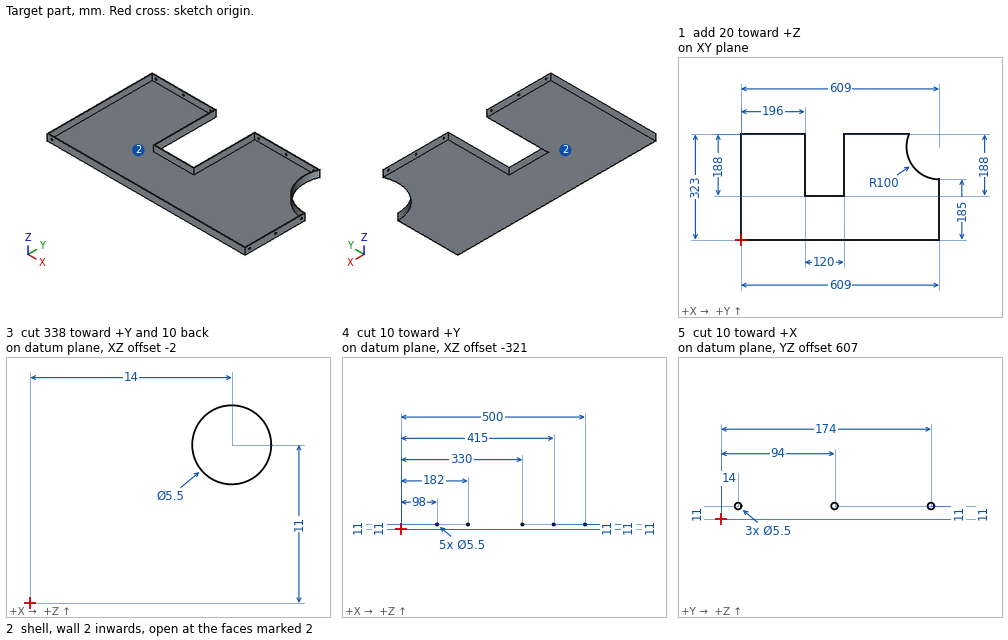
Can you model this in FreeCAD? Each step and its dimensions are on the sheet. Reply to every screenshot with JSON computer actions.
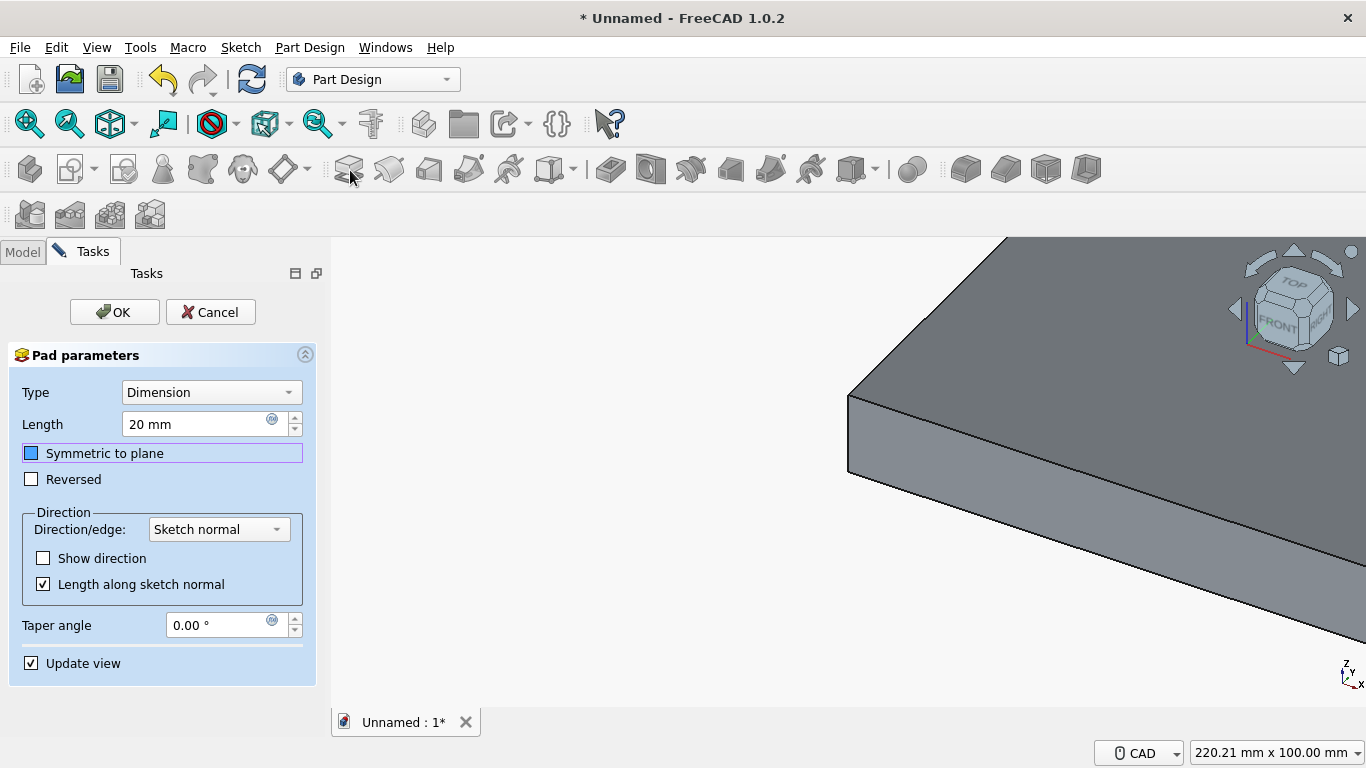
{"action": "left_click", "coordinate": [115, 312]}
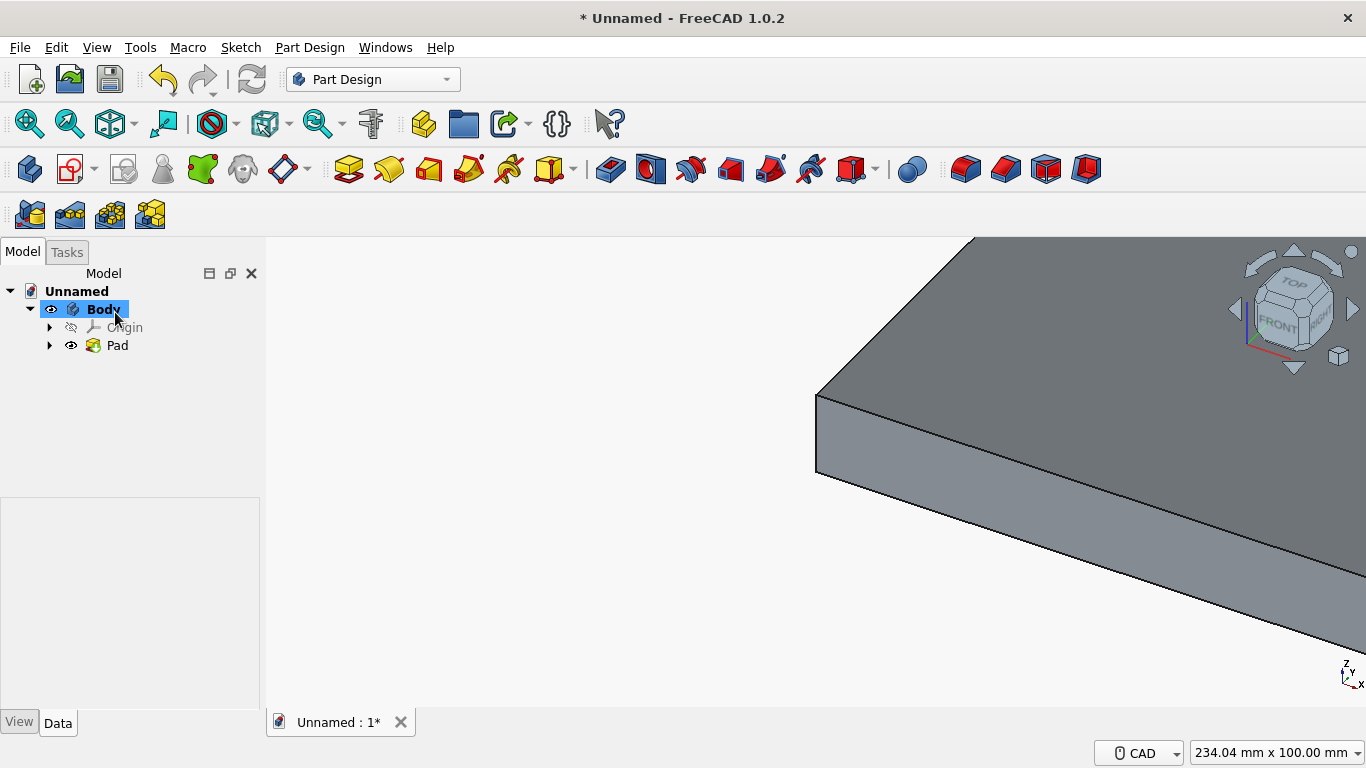
{"action": "left_click", "coordinate": [30, 124]}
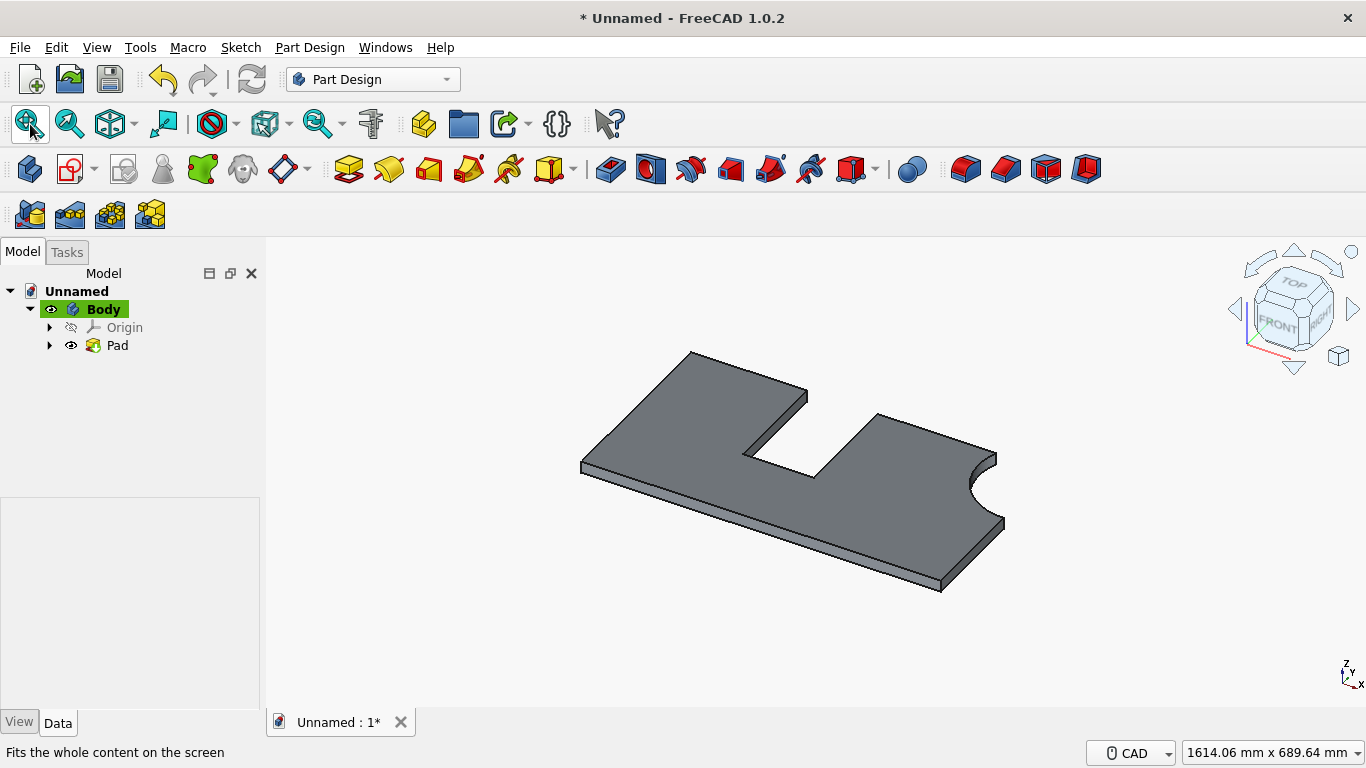
{"action": "left_click", "coordinate": [903, 515]}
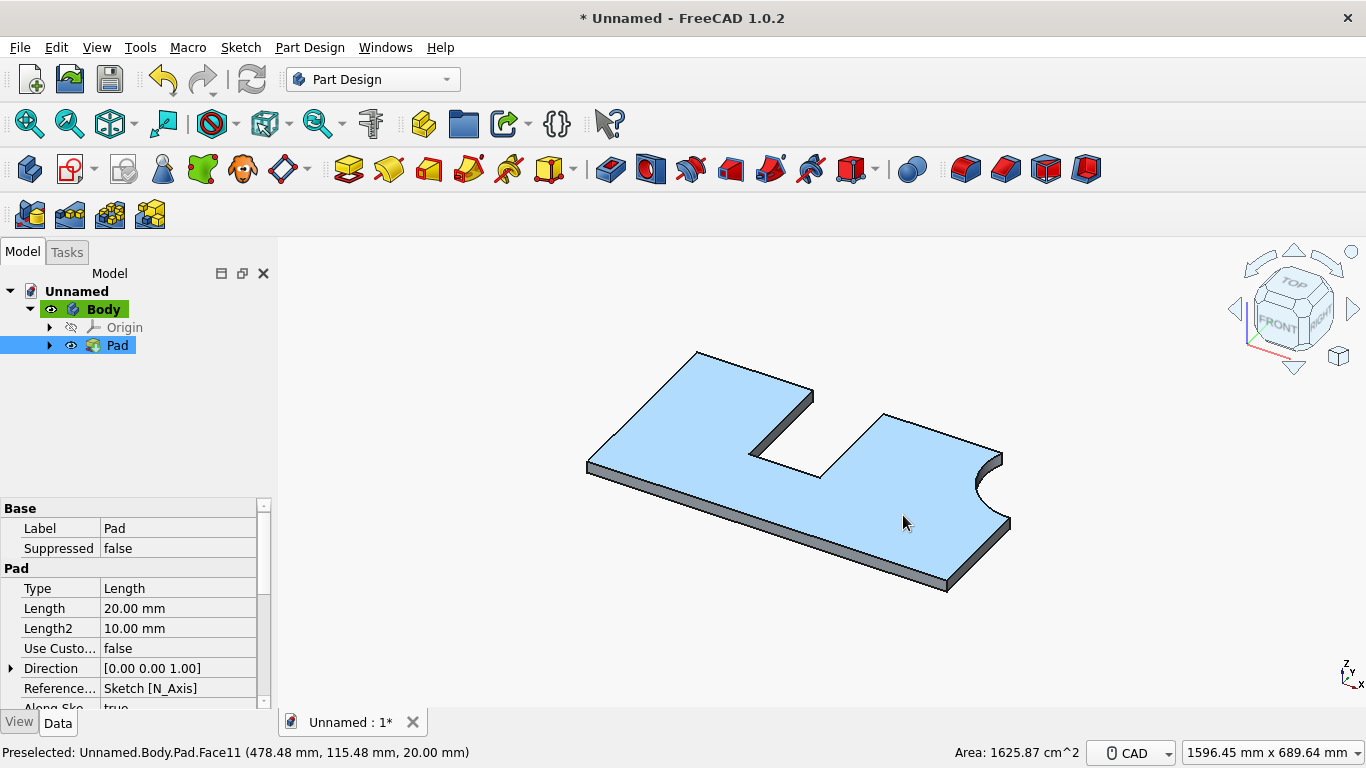
{"action": "left_click", "coordinate": [1086, 170]}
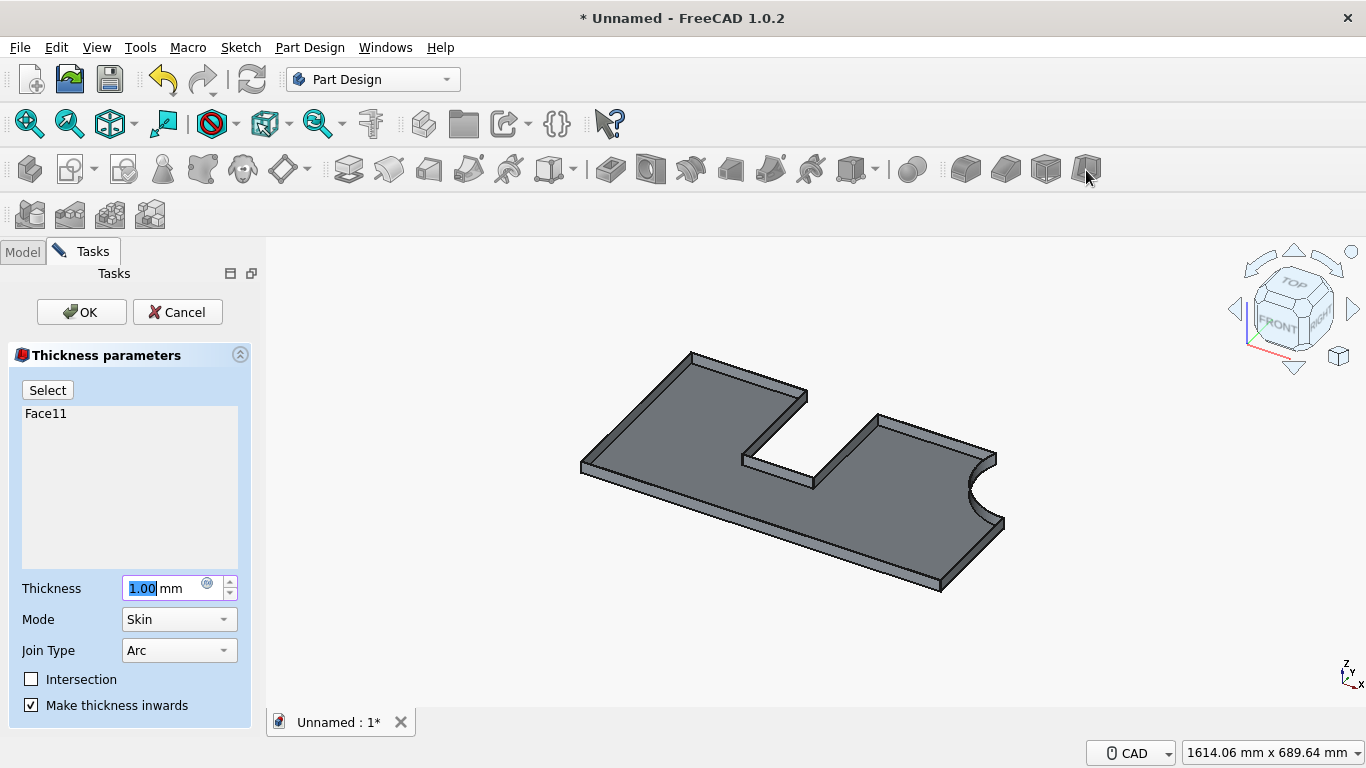
{"action": "type", "text": "2"}
{"action": "key", "text": "Tab"}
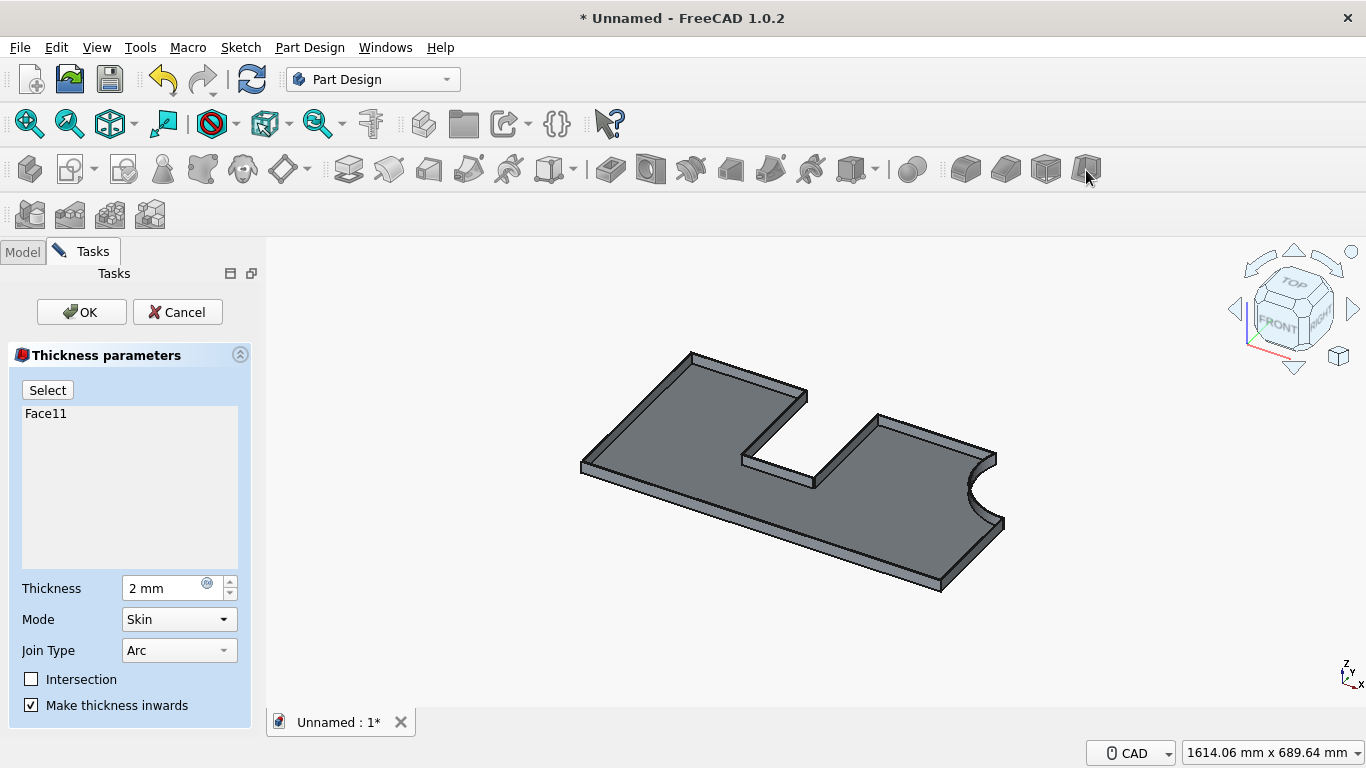
{"action": "left_click", "coordinate": [180, 650]}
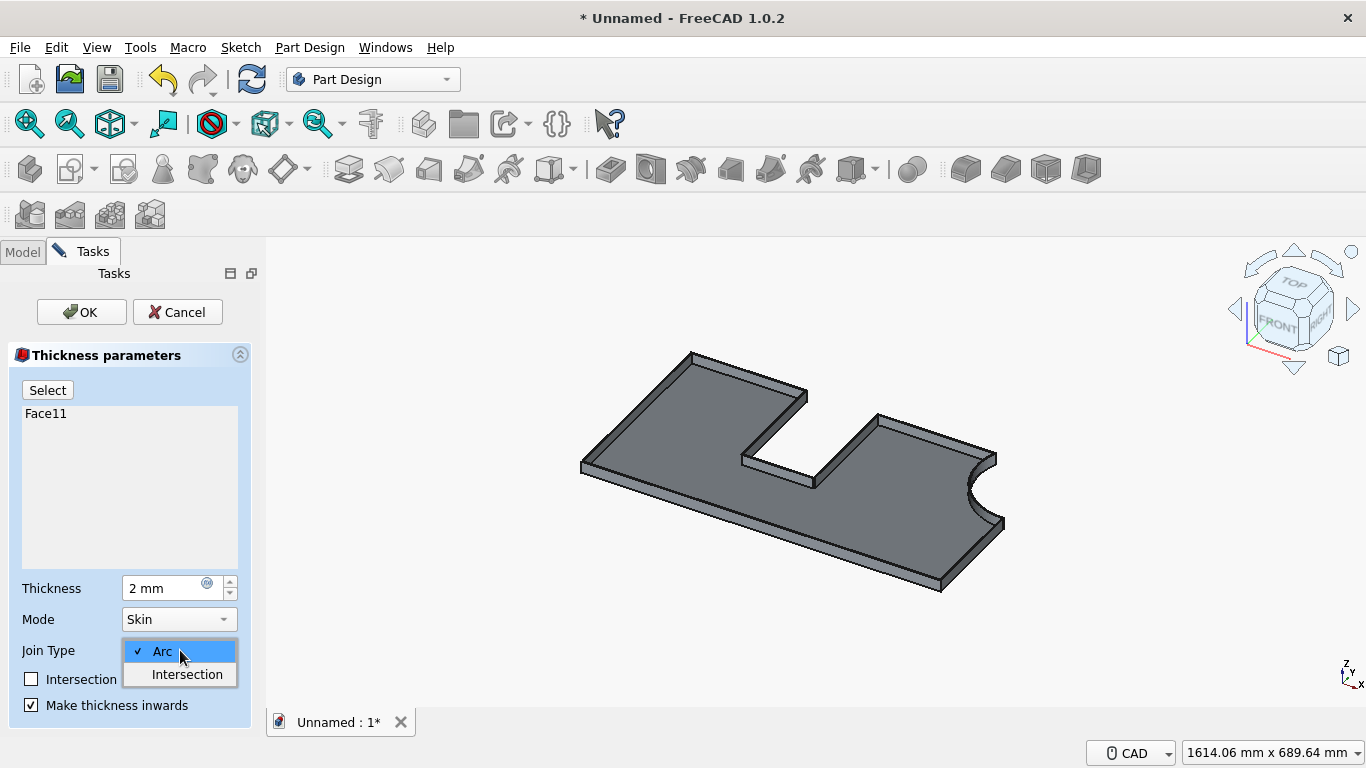
{"action": "left_click", "coordinate": [179, 674]}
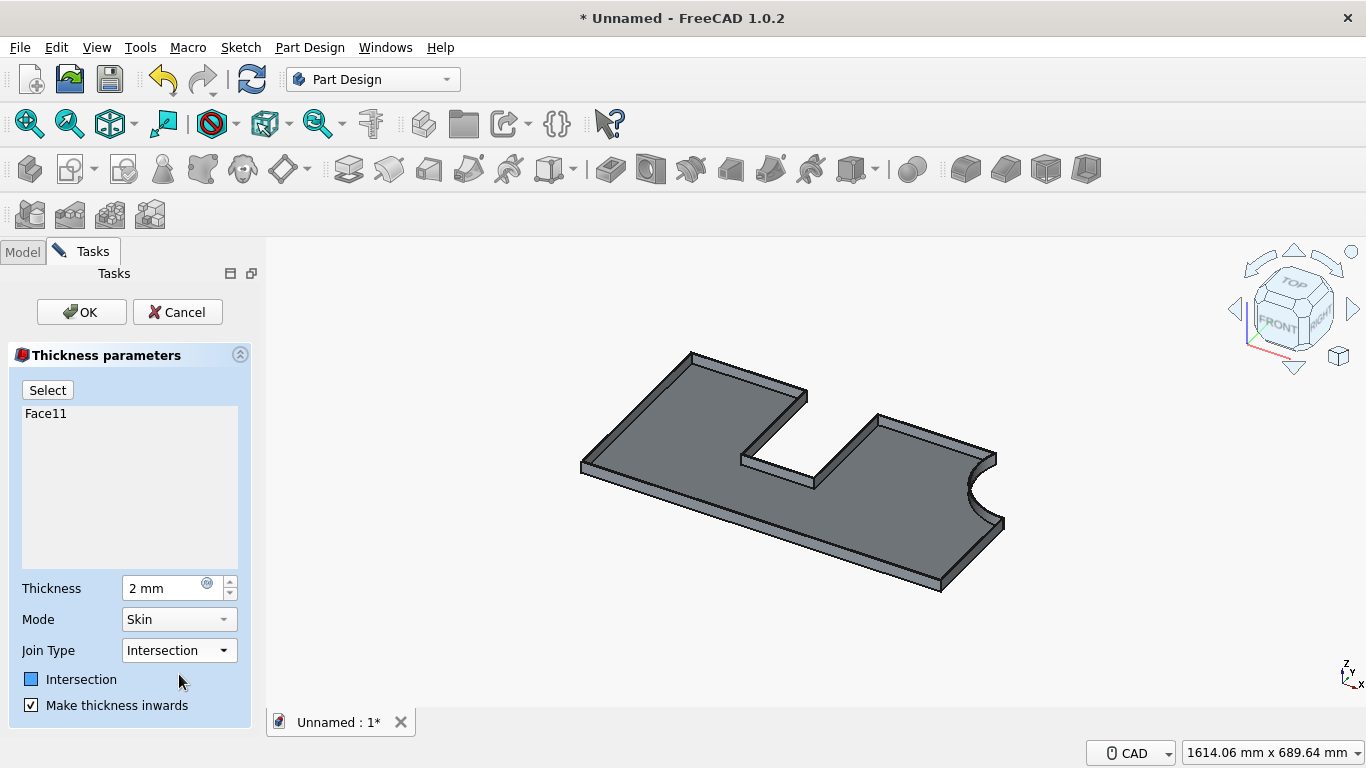
{"action": "left_click", "coordinate": [82, 312]}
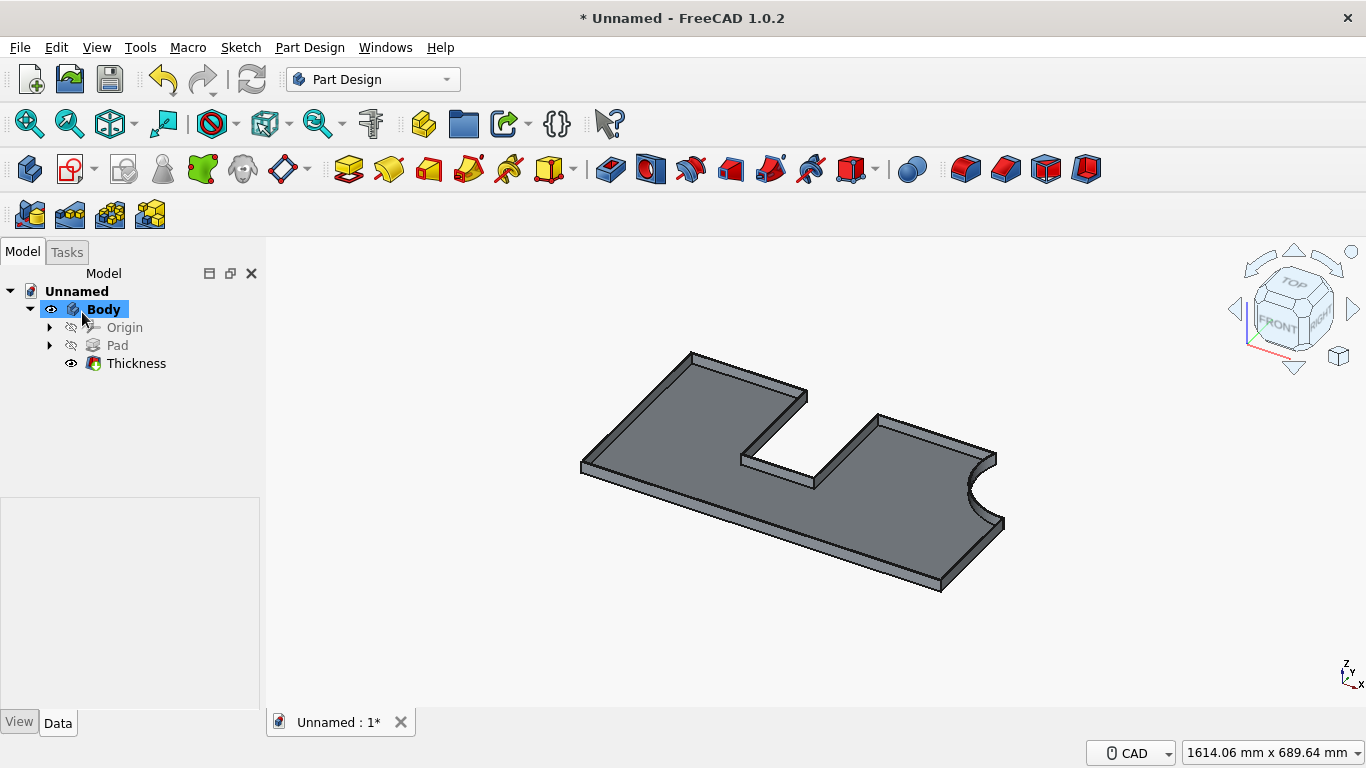
{"action": "left_click", "coordinate": [50, 327]}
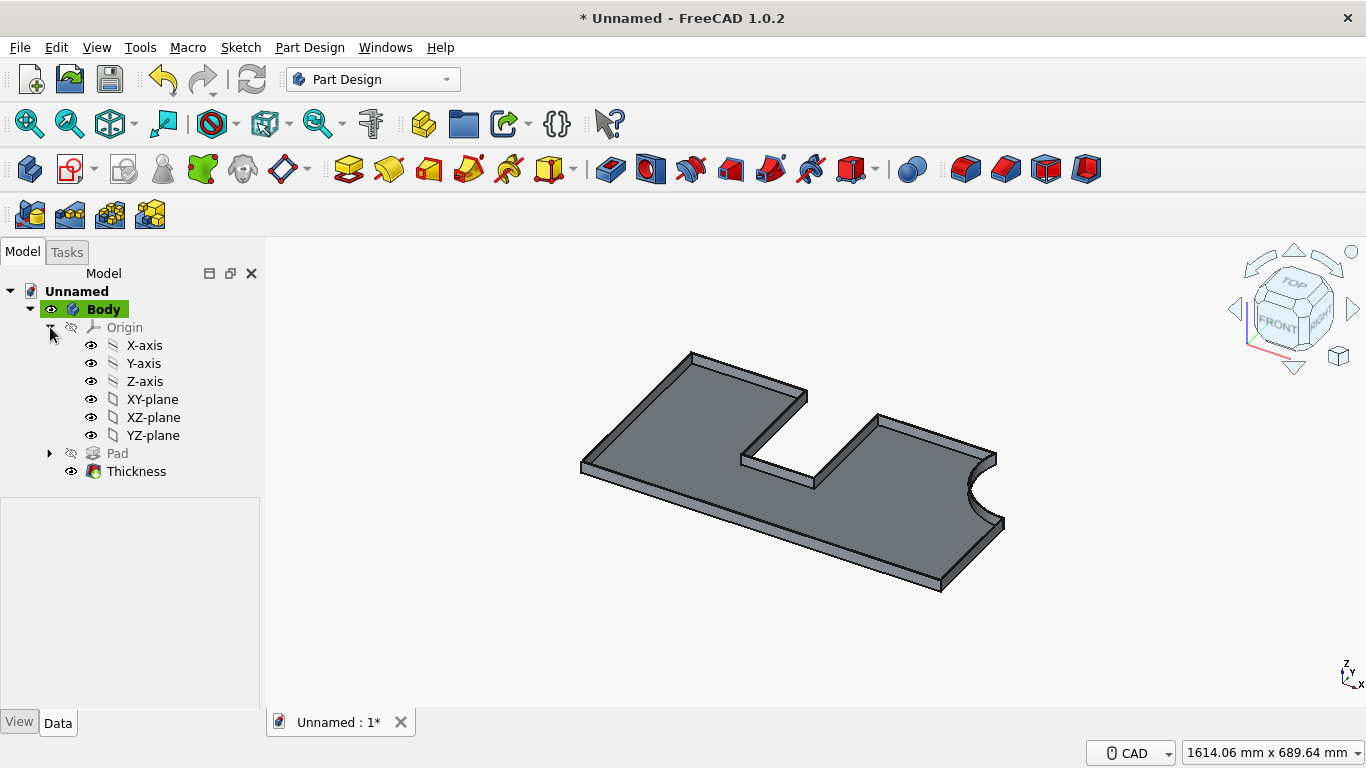
{"action": "left_click", "coordinate": [136, 417]}